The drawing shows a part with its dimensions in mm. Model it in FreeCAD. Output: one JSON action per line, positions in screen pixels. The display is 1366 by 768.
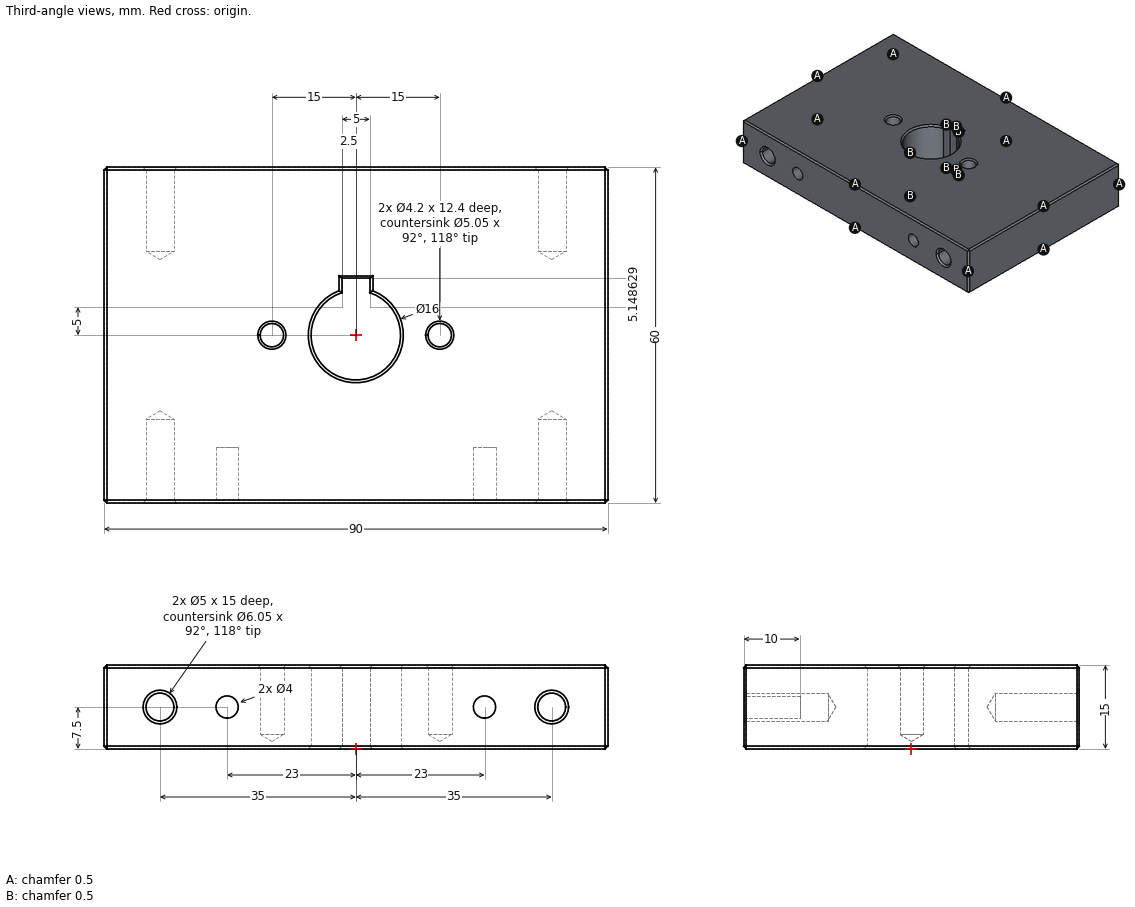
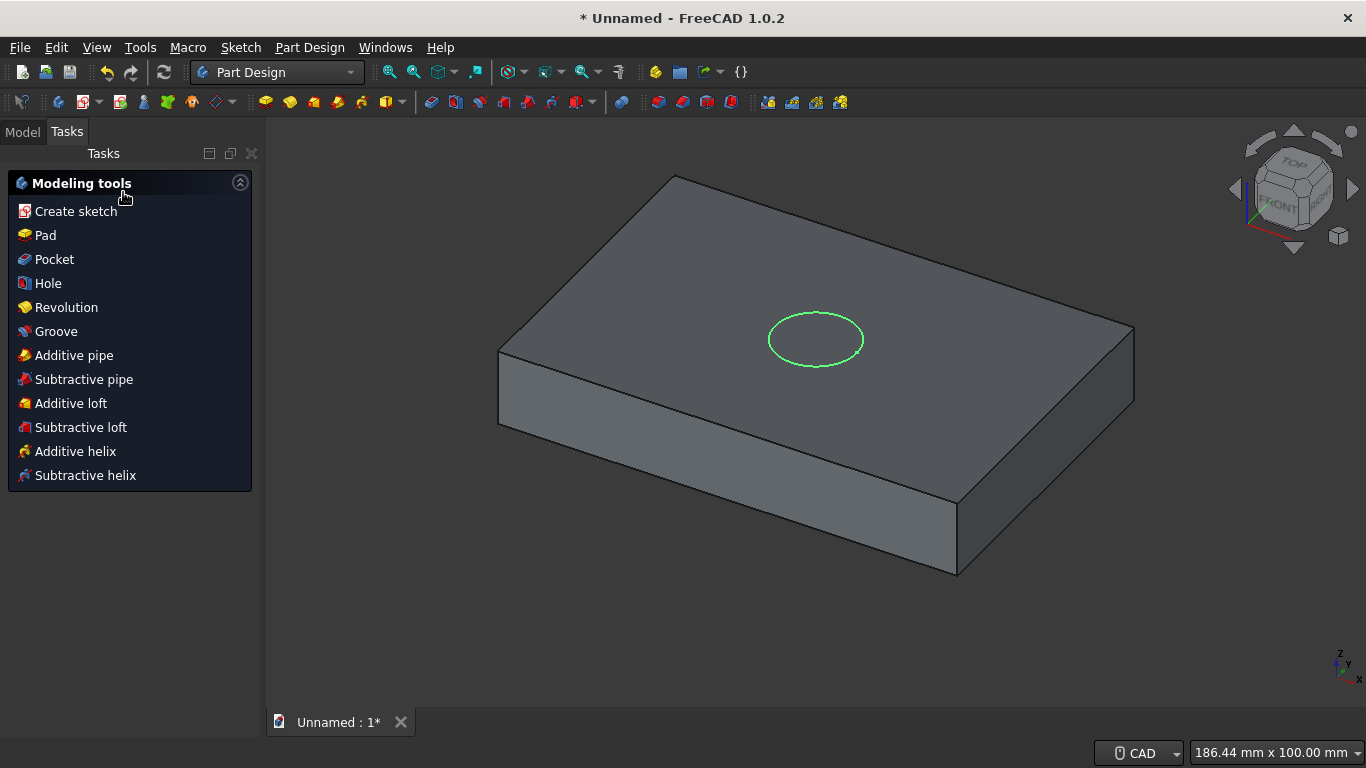
{"action": "left_click", "coordinate": [432, 102]}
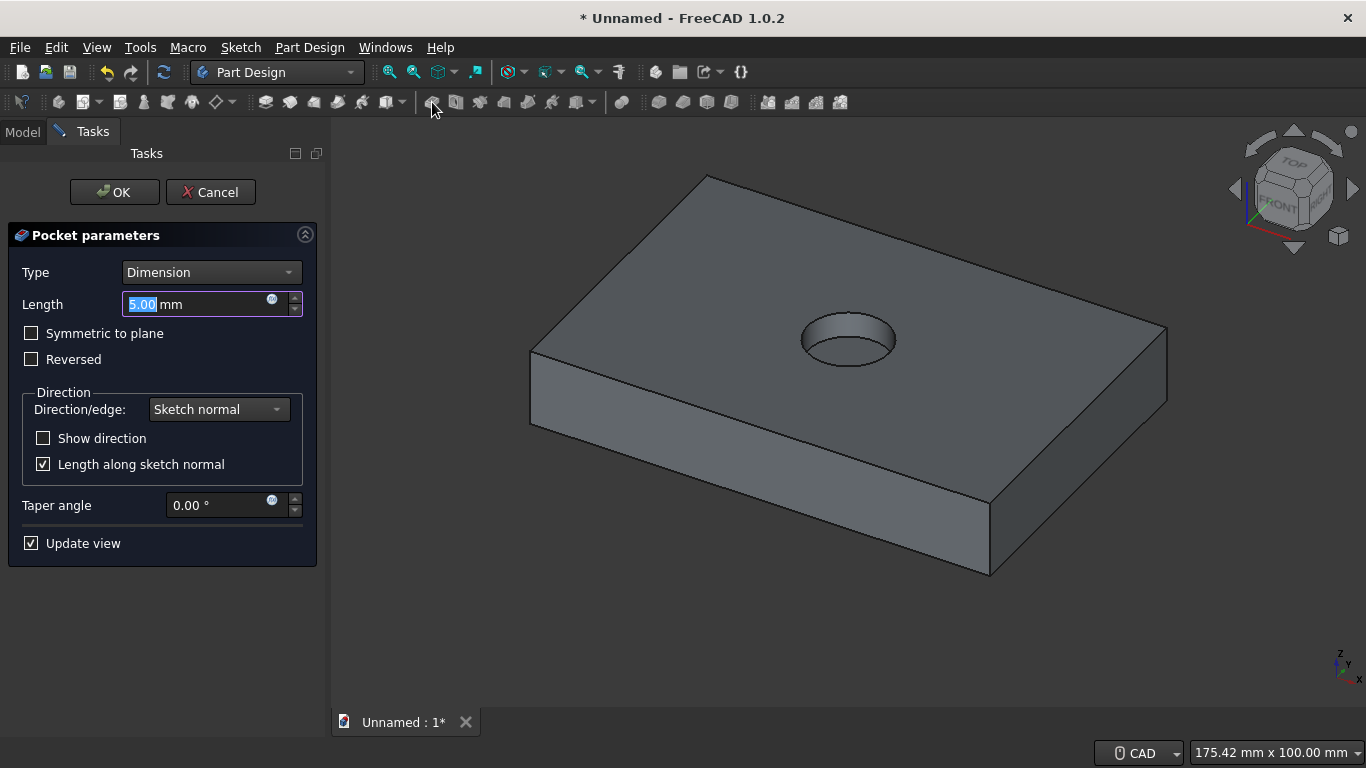
{"action": "left_click", "coordinate": [212, 272]}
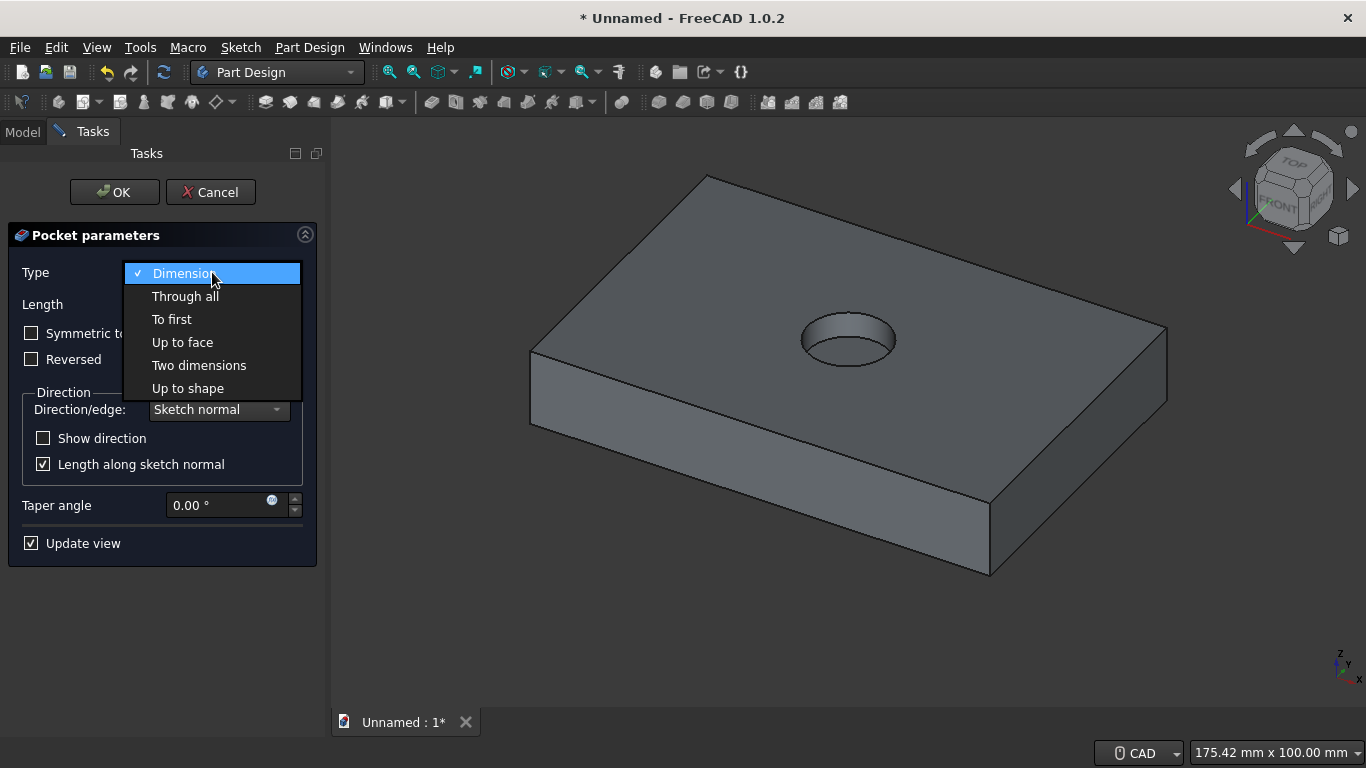
{"action": "left_click", "coordinate": [212, 296]}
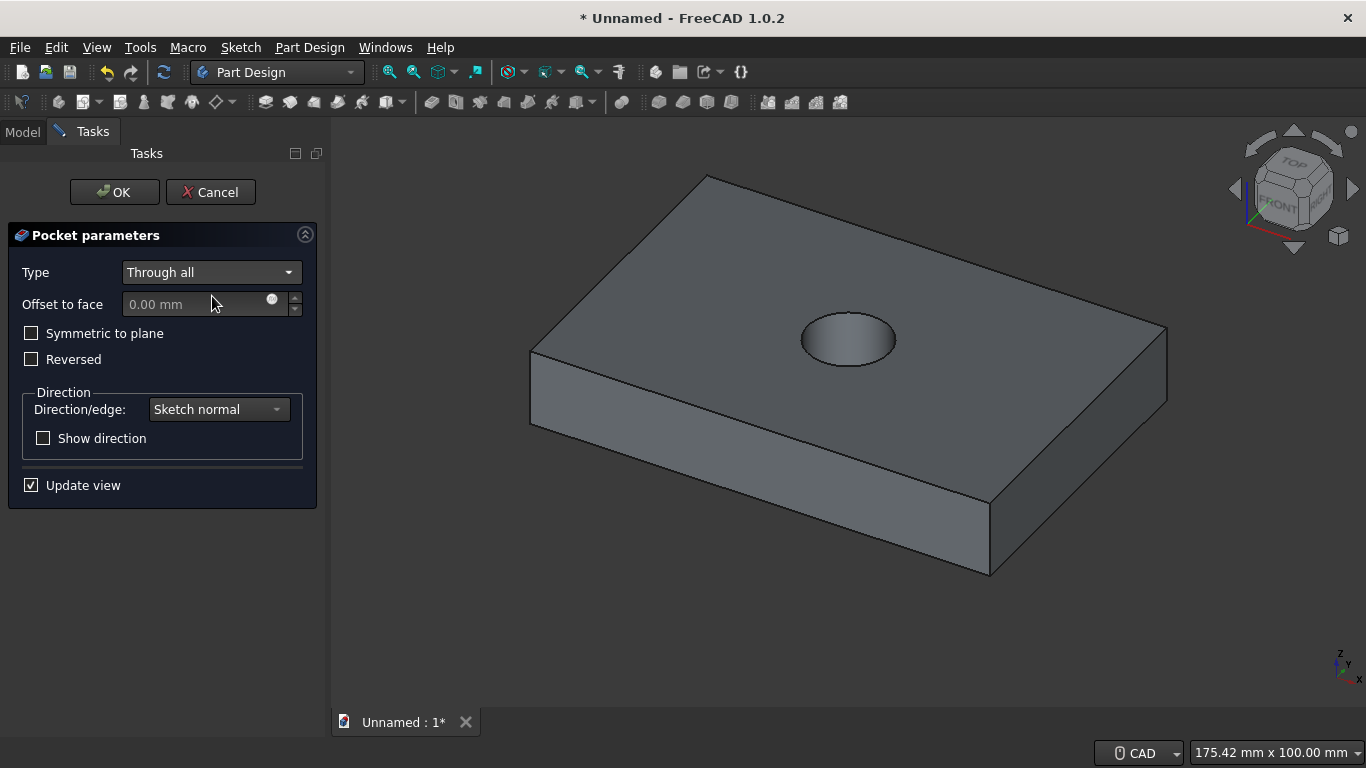
{"action": "left_click", "coordinate": [115, 192]}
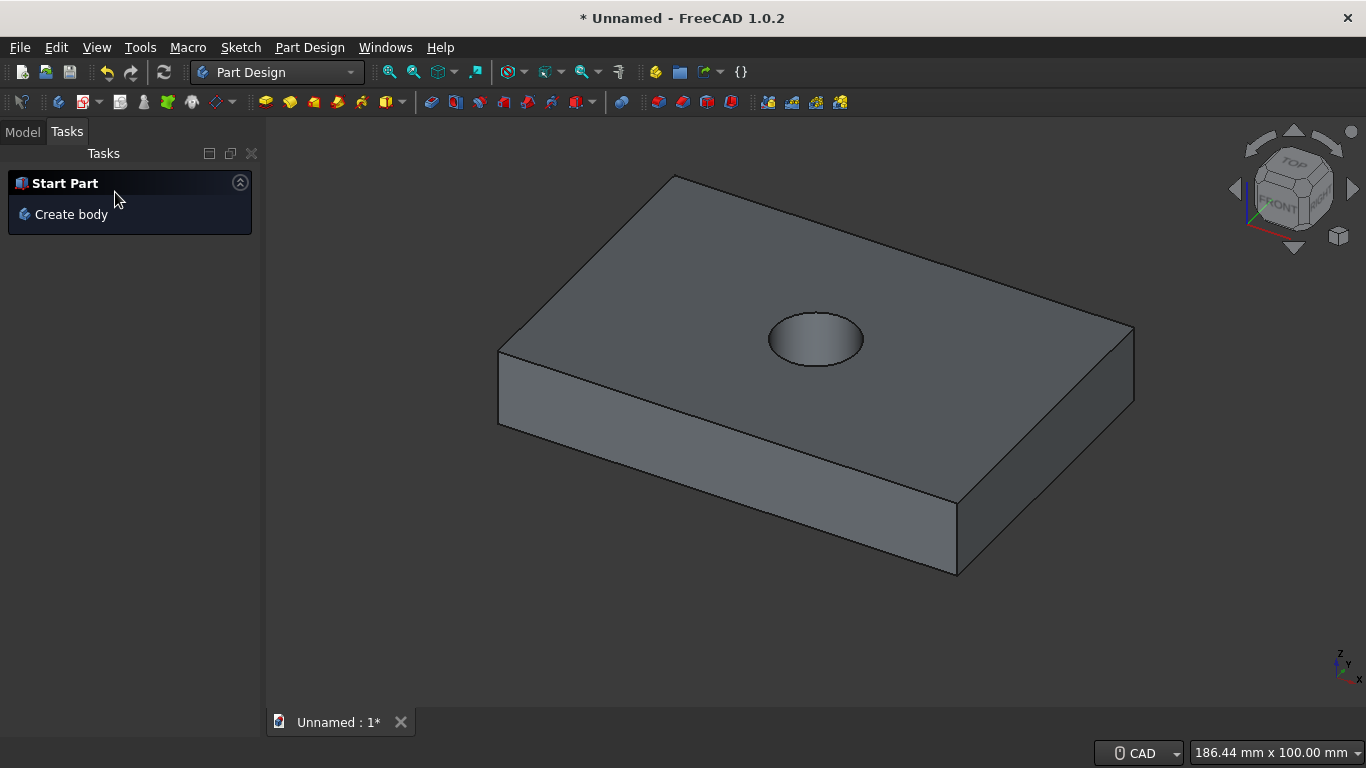
{"action": "left_click", "coordinate": [710, 270]}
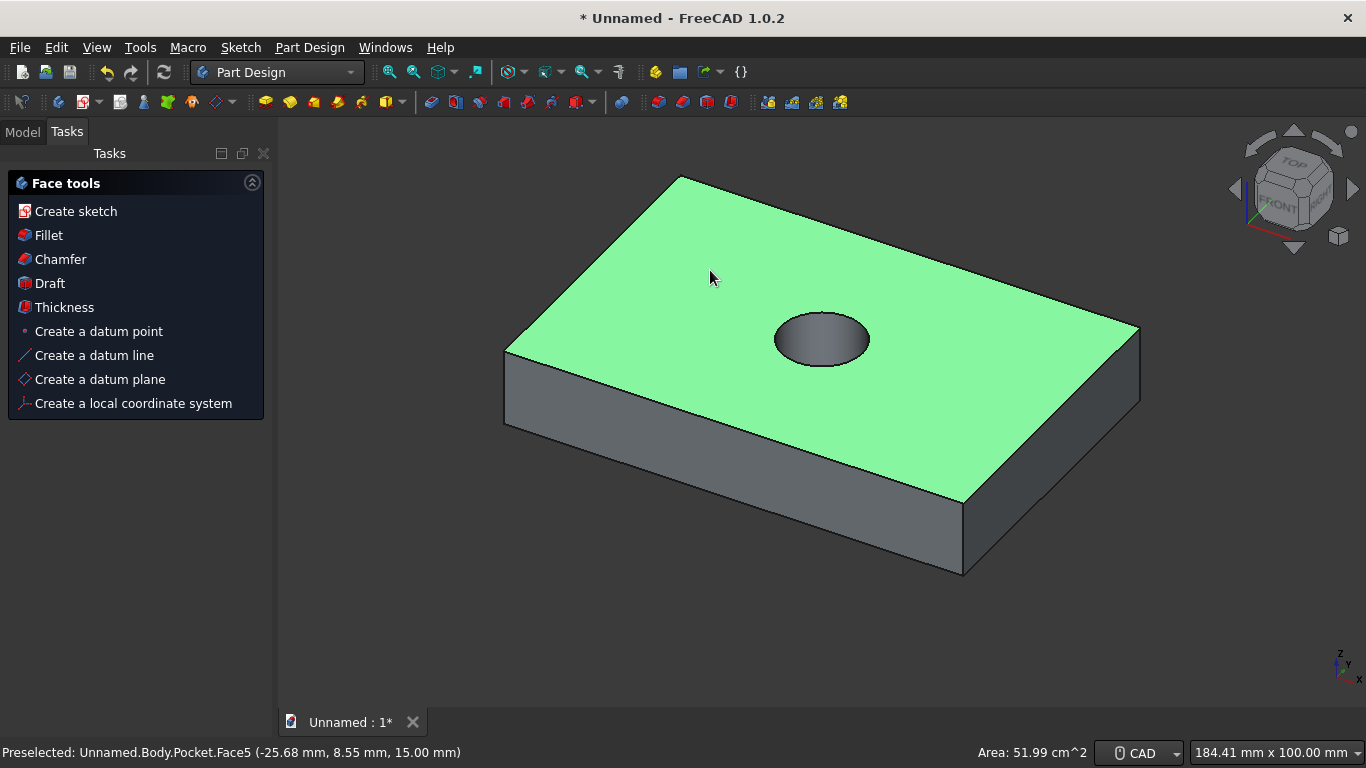
{"action": "left_click", "coordinate": [84, 102]}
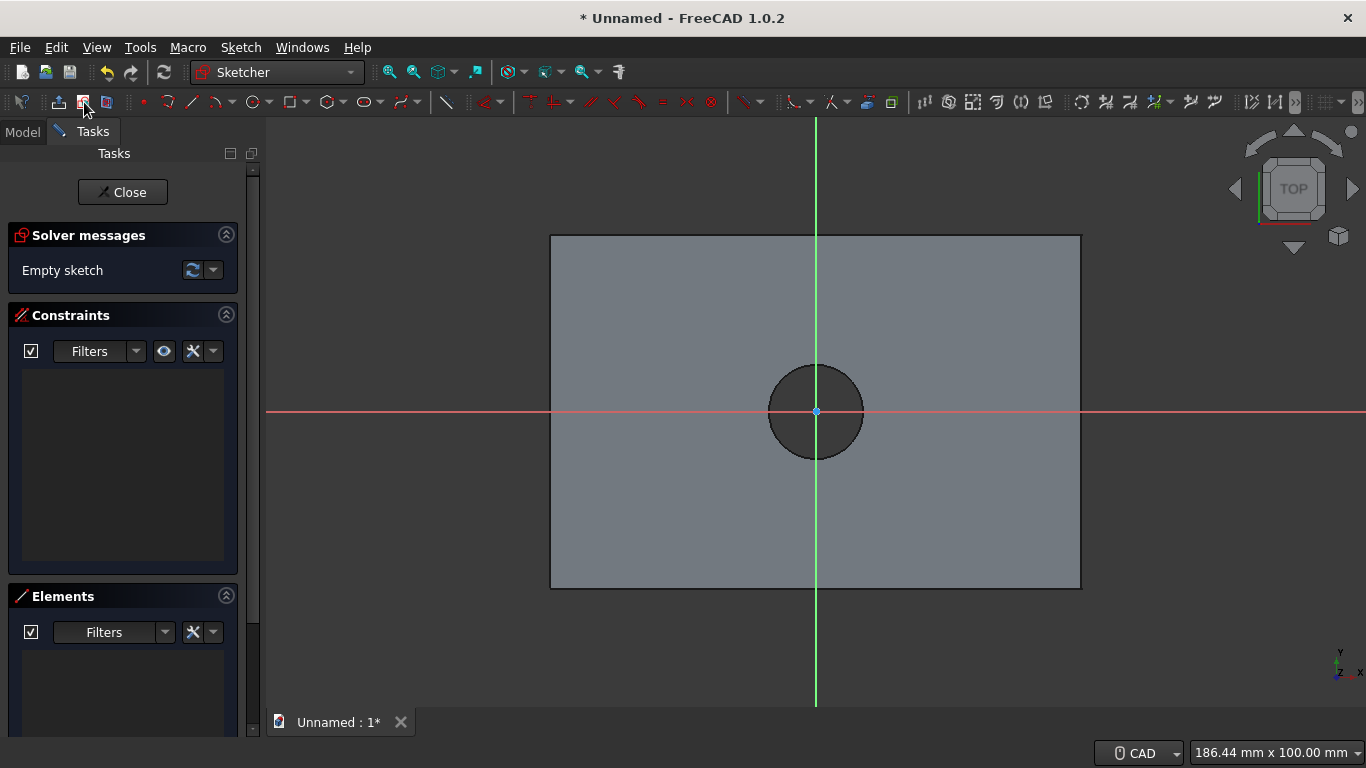
{"action": "scroll", "coordinate": [830, 376], "scroll_direction": "up", "scroll_amount": 9}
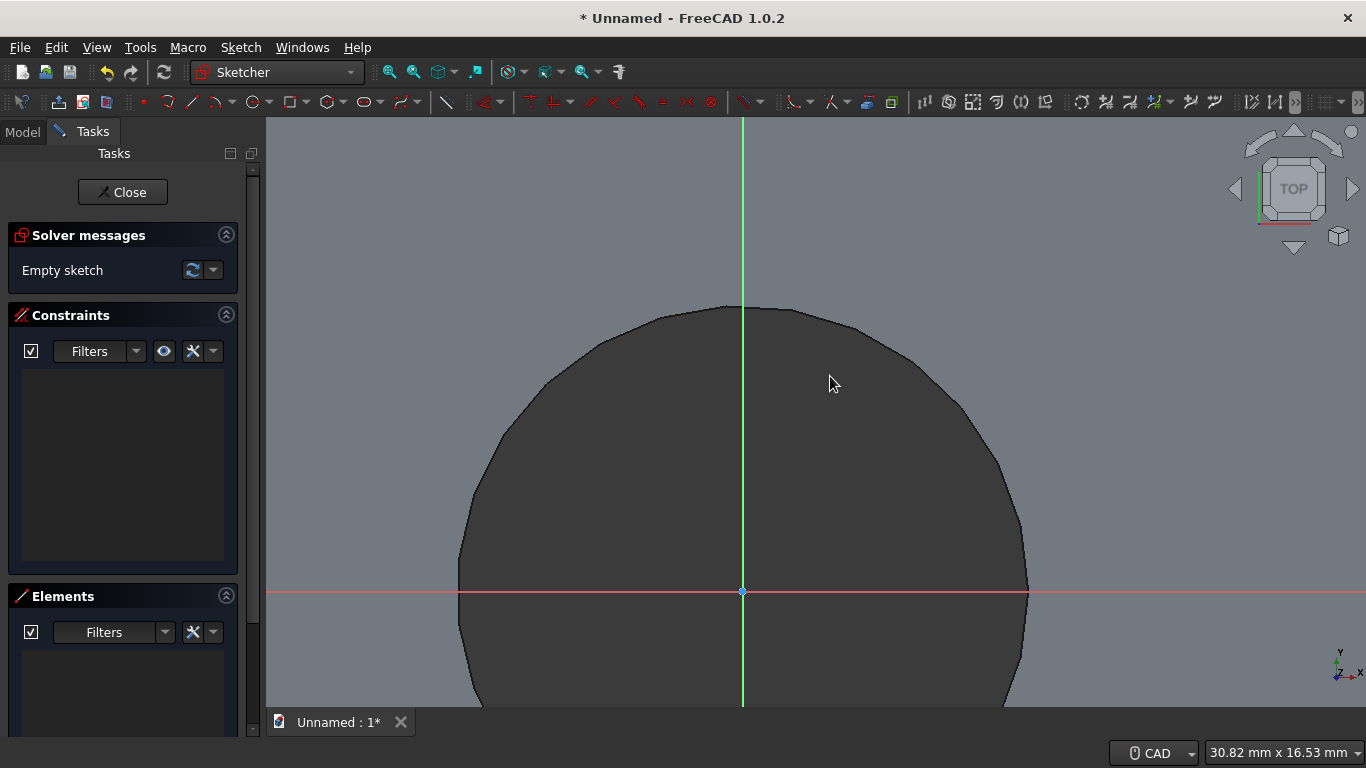
{"action": "key", "text": "g r"}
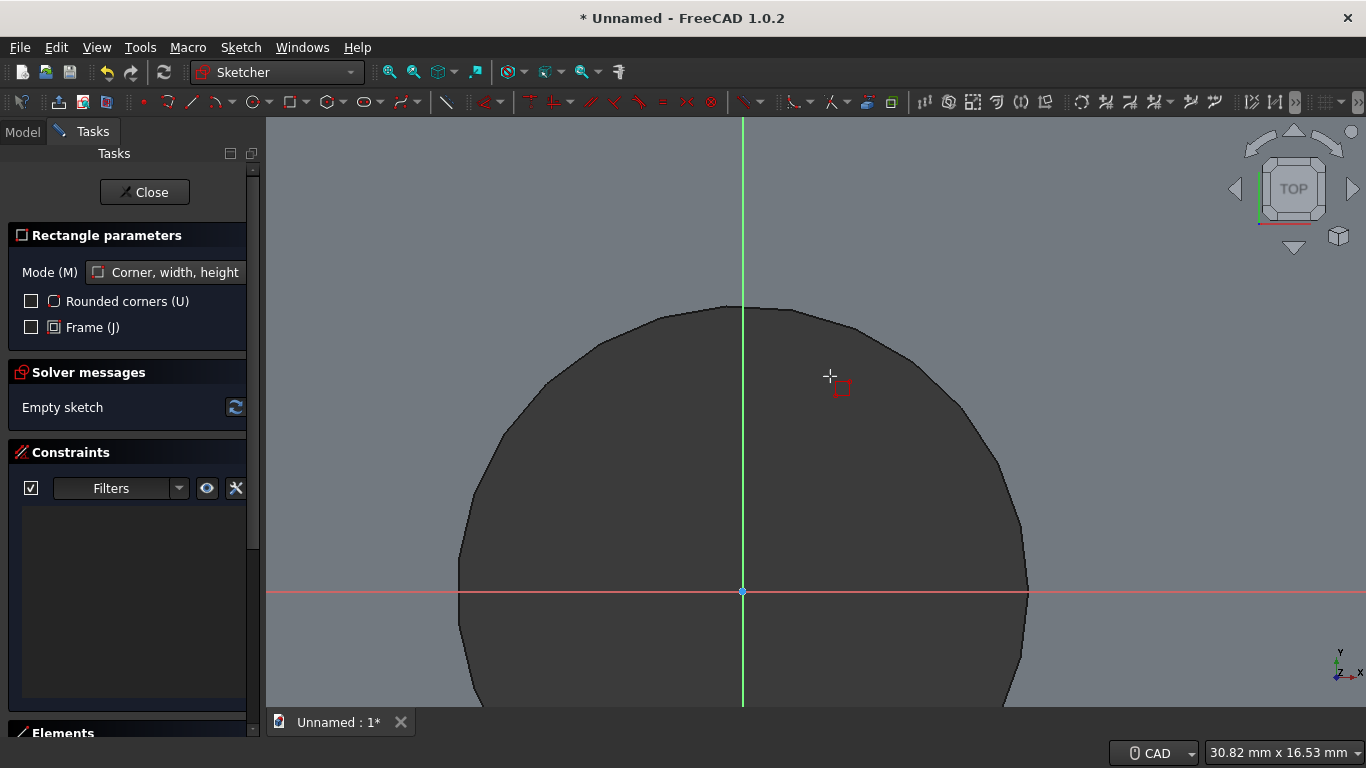
{"action": "left_click", "coordinate": [653, 229]}
{"action": "mouse_move", "coordinate": [832, 413]}